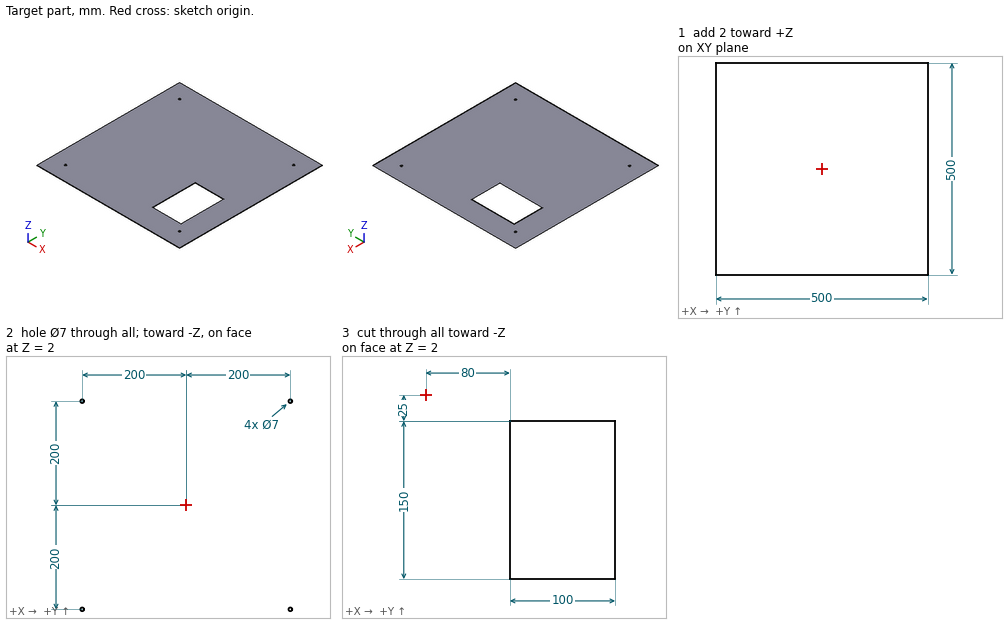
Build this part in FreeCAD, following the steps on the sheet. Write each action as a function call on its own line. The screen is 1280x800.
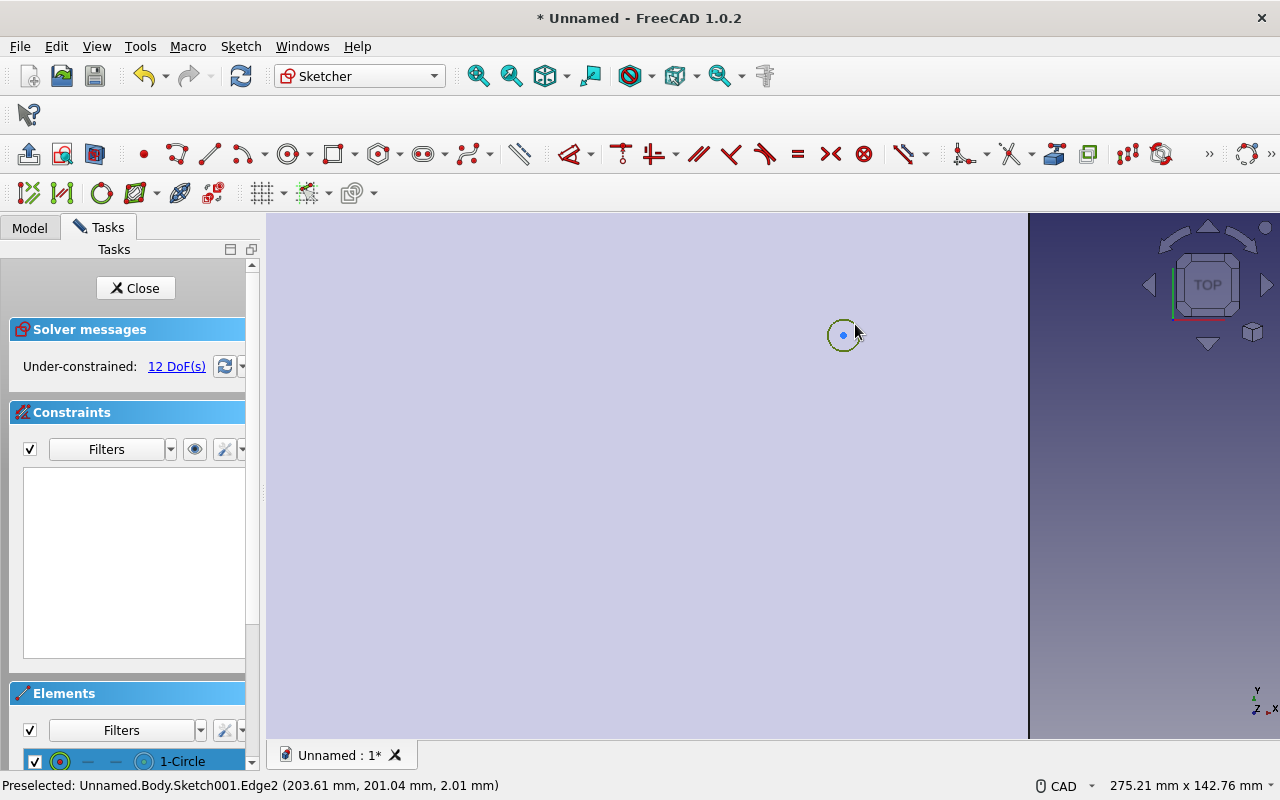
scroll(856, 326, down, 8)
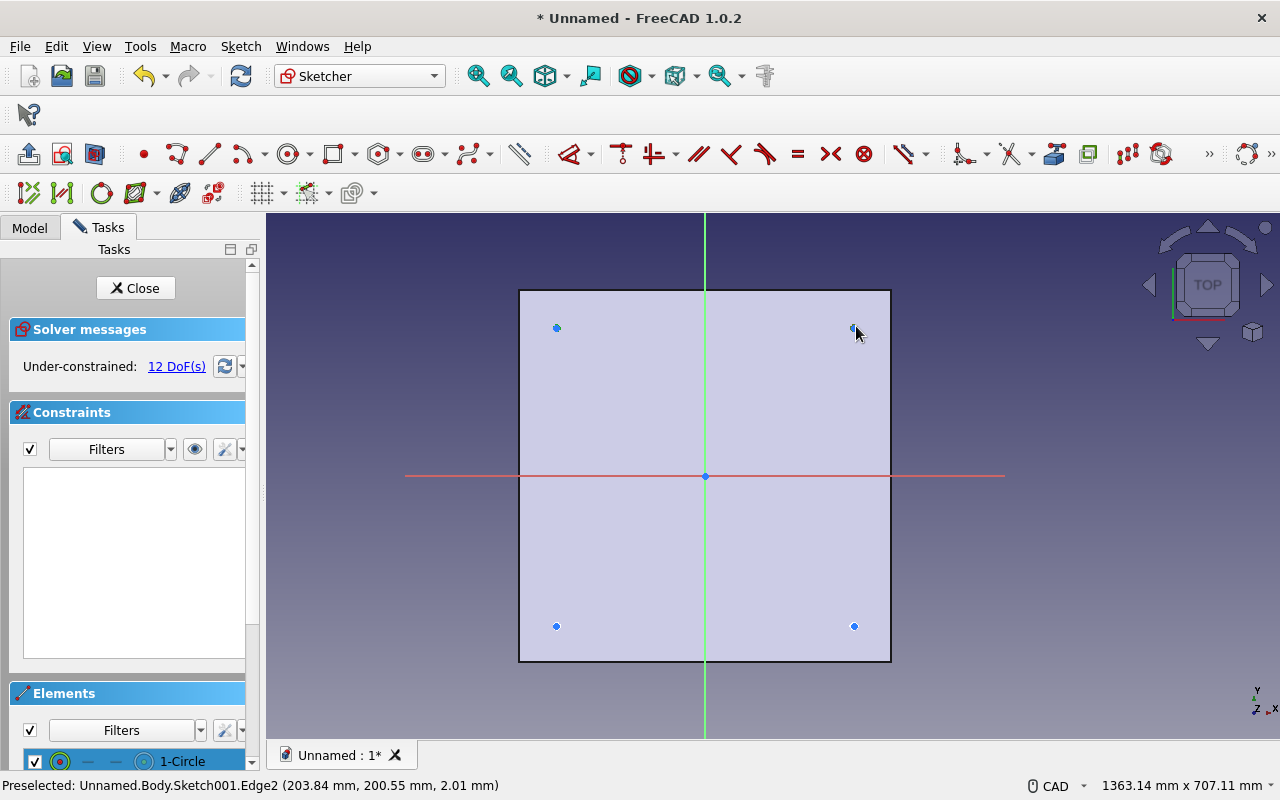
scroll(559, 624, up, 8)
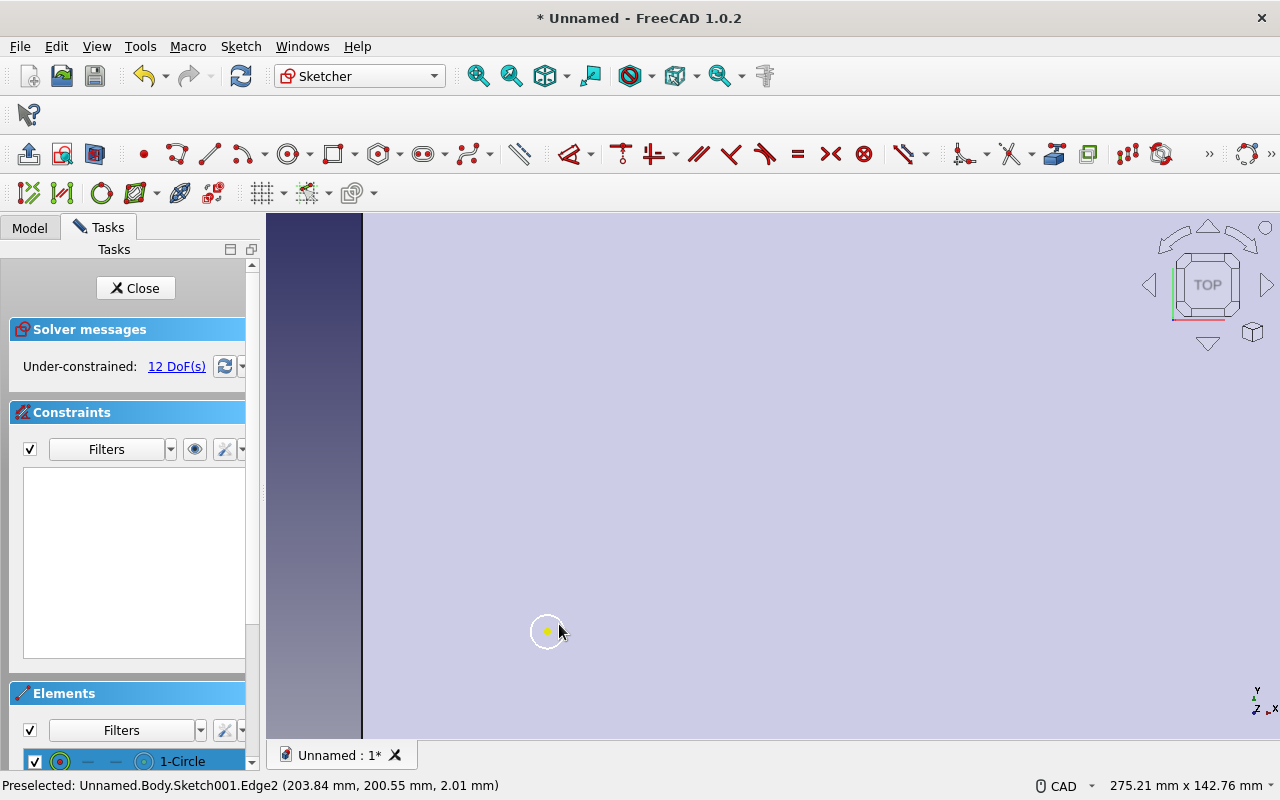
click(559, 620)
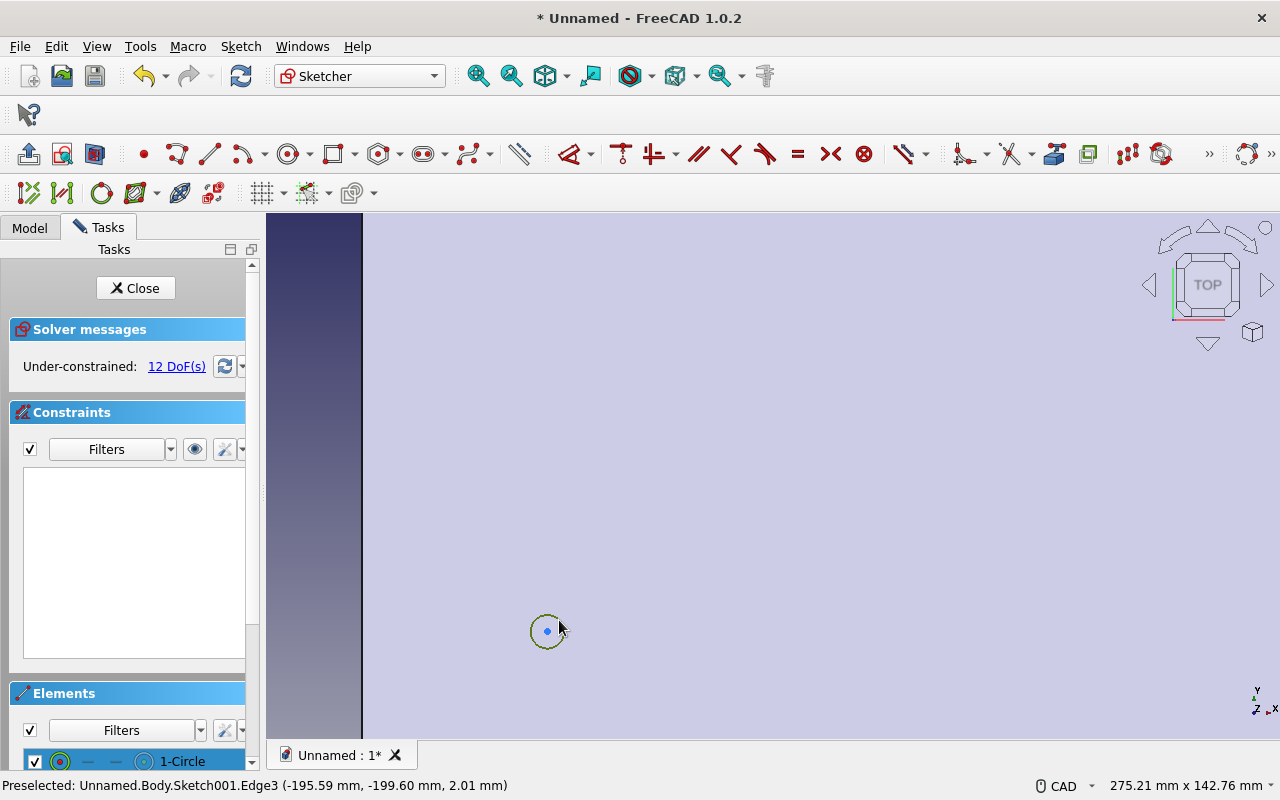
scroll(558, 625, down, 8)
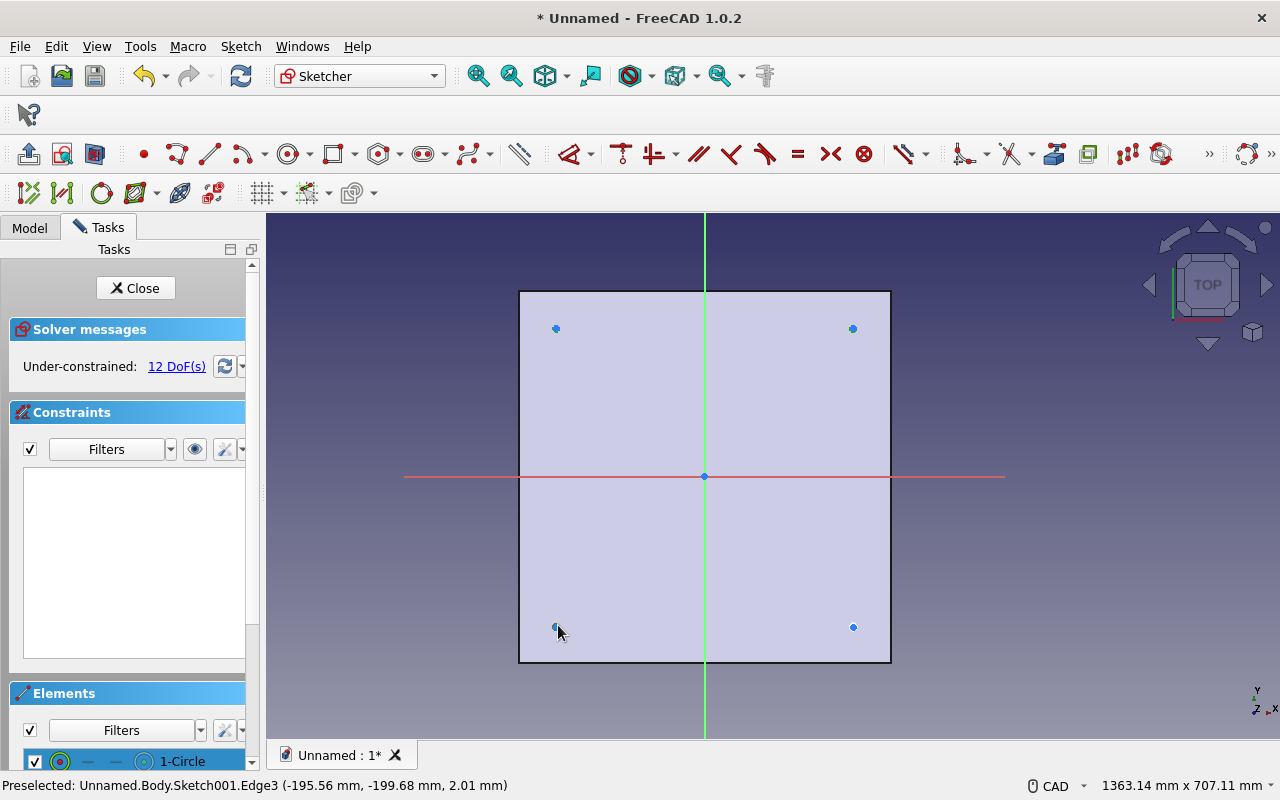
scroll(856, 624, up, 7)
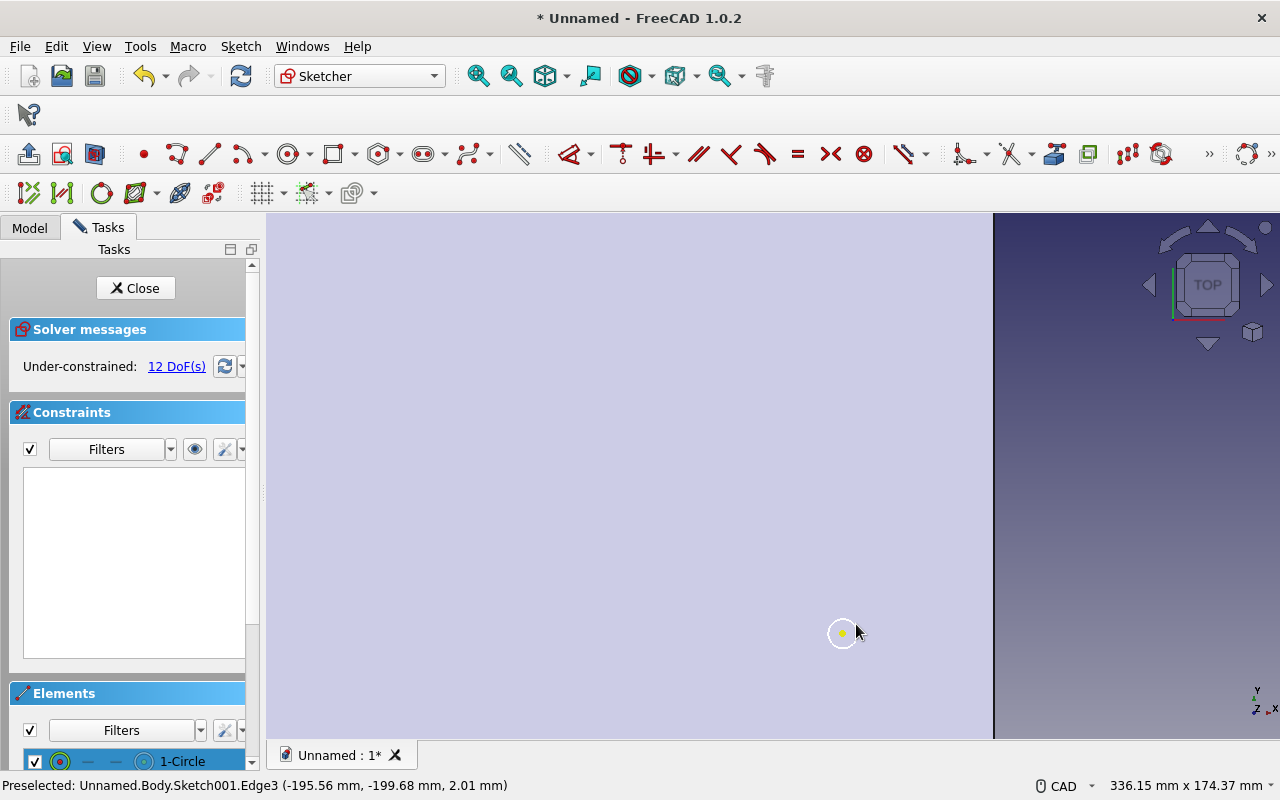
click(853, 623)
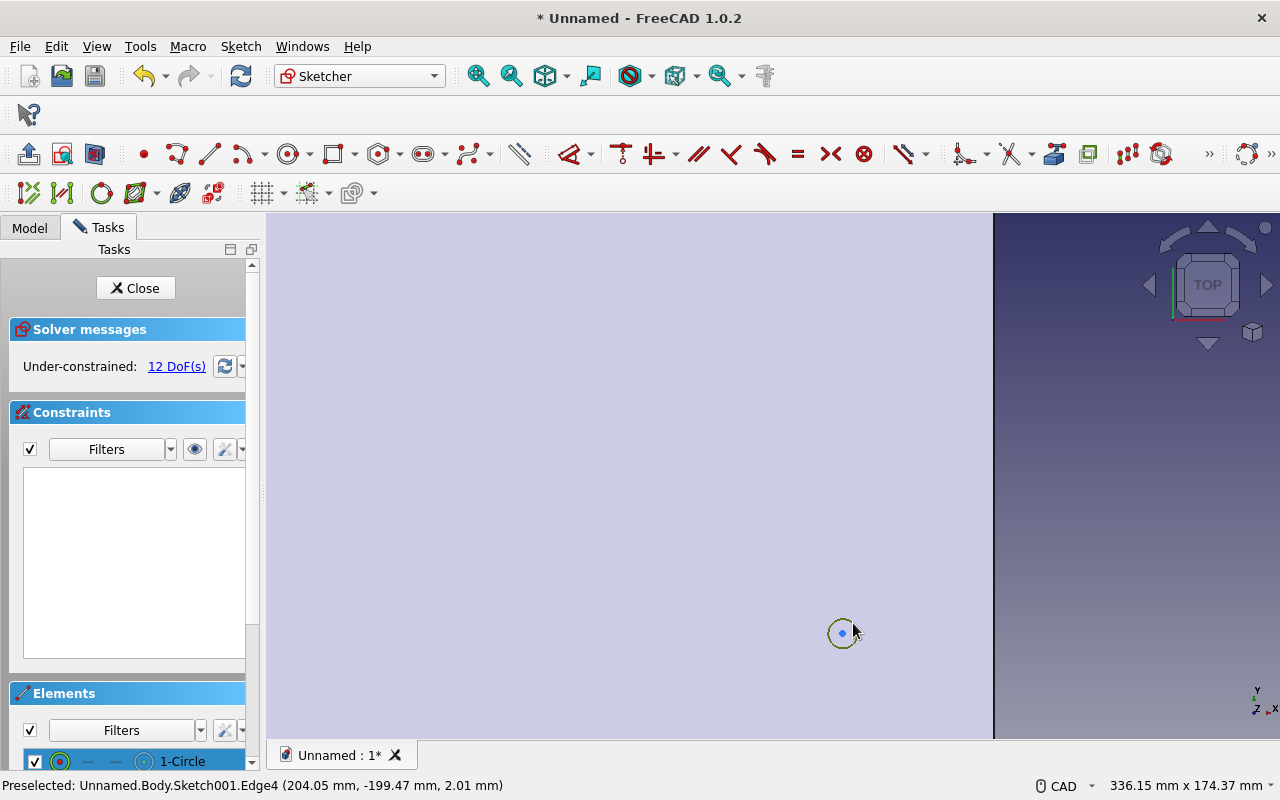
key(e)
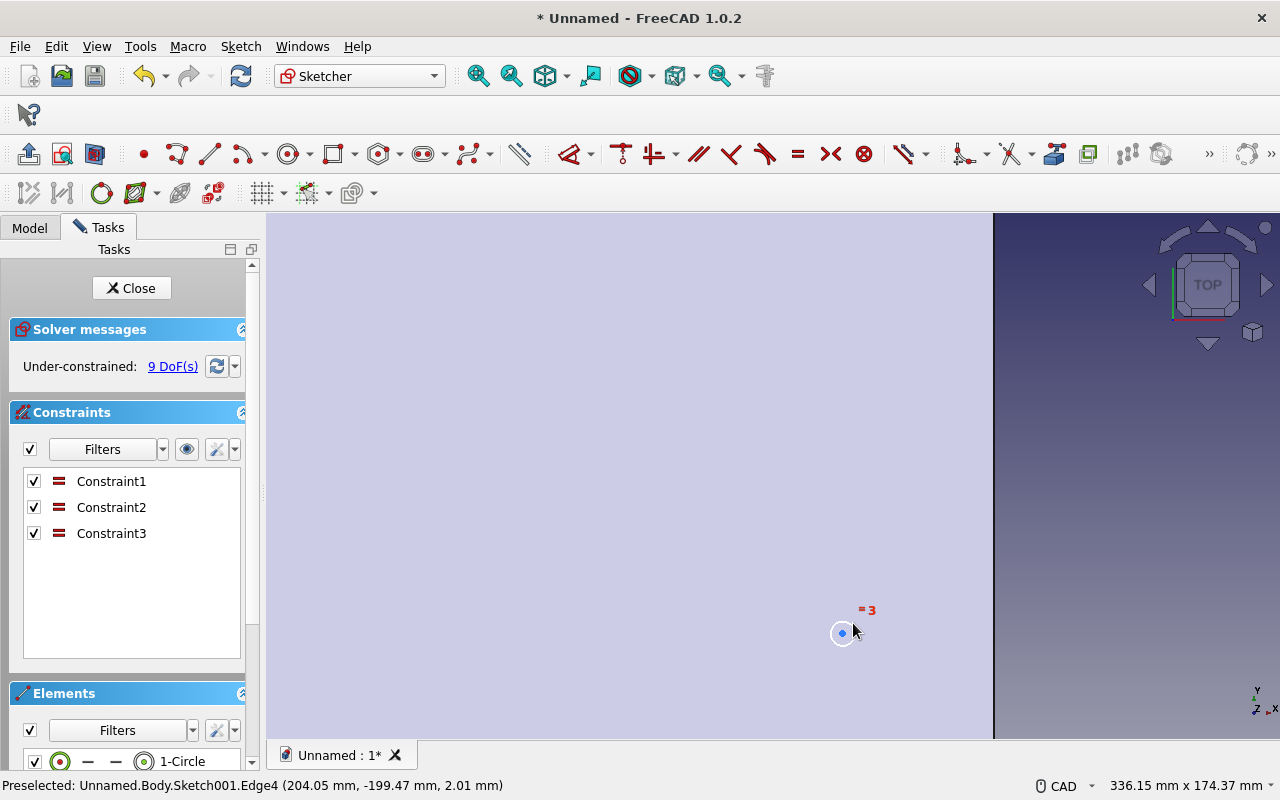
scroll(857, 624, down, 7)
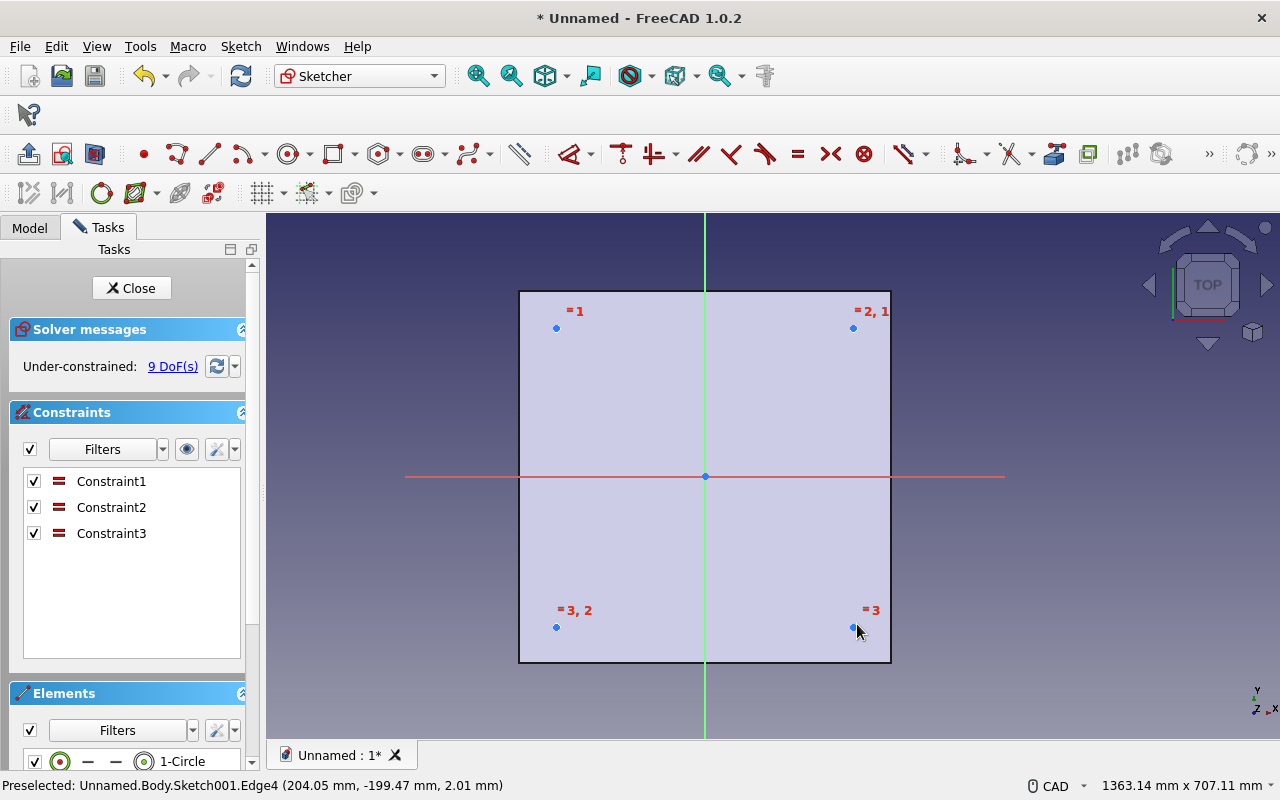
click(557, 329)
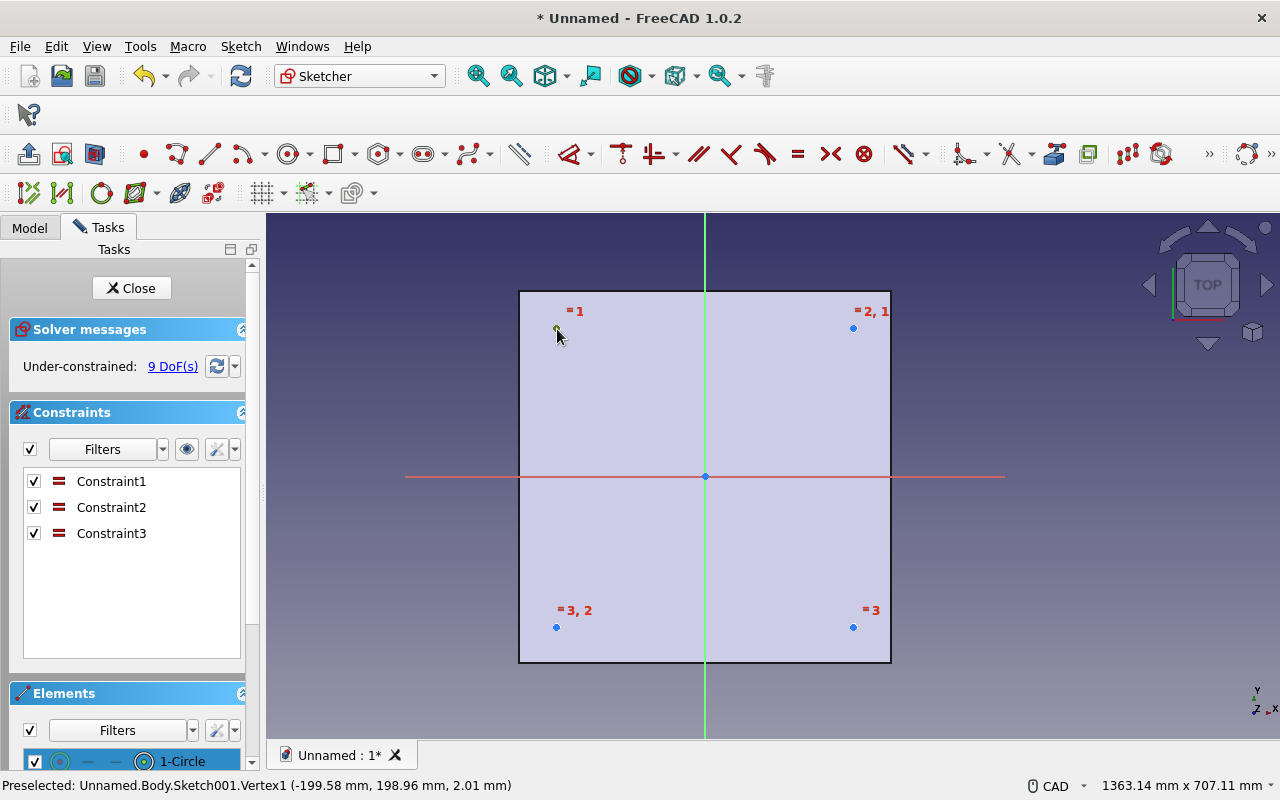
click(854, 329)